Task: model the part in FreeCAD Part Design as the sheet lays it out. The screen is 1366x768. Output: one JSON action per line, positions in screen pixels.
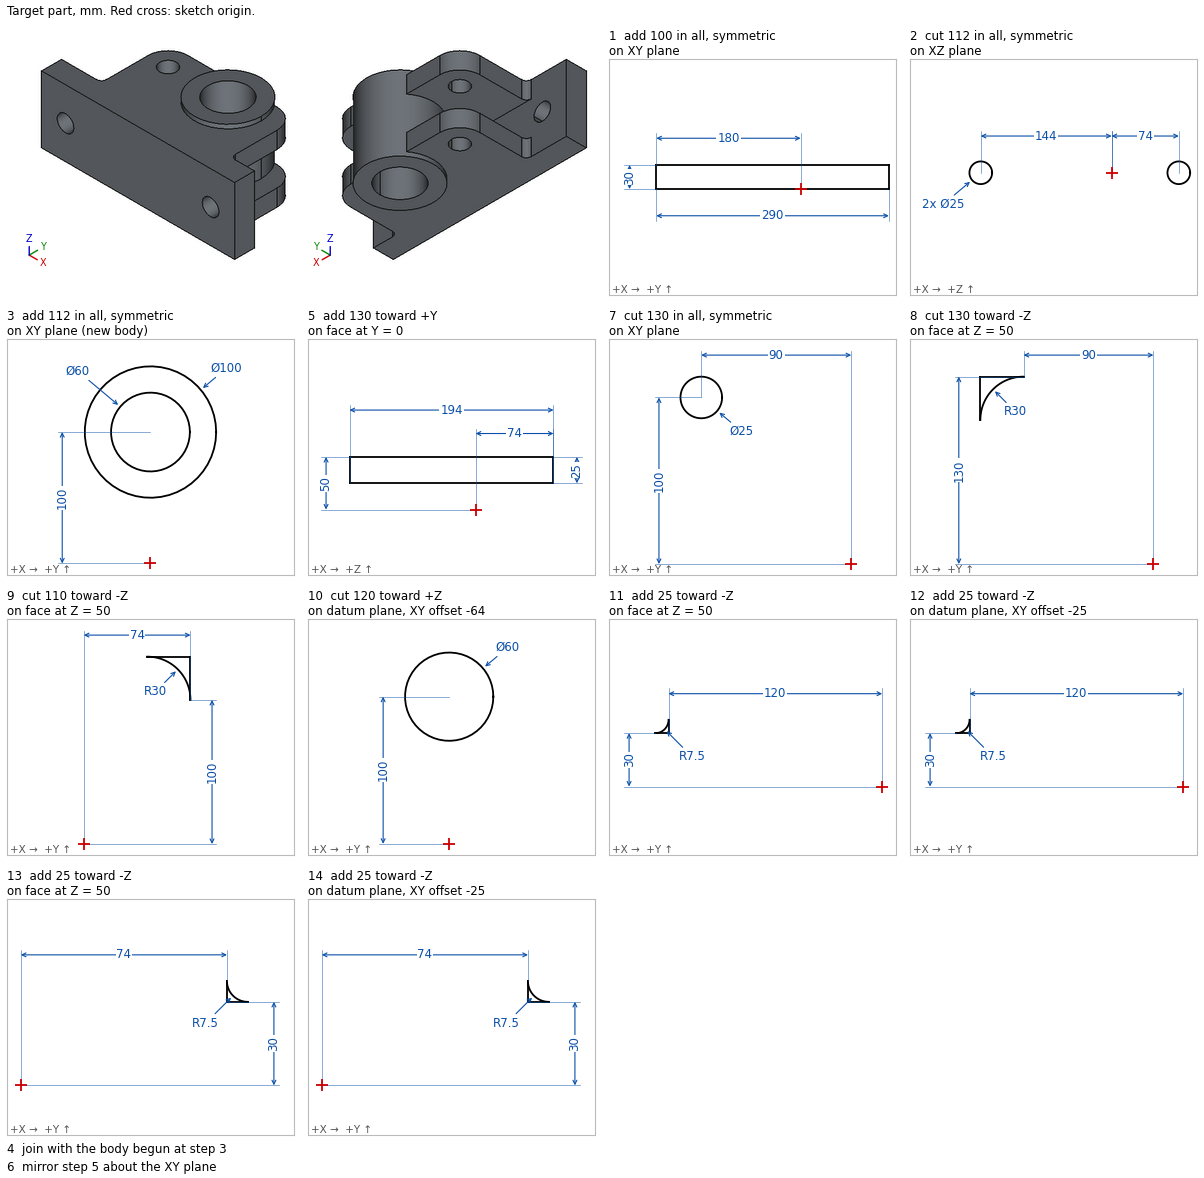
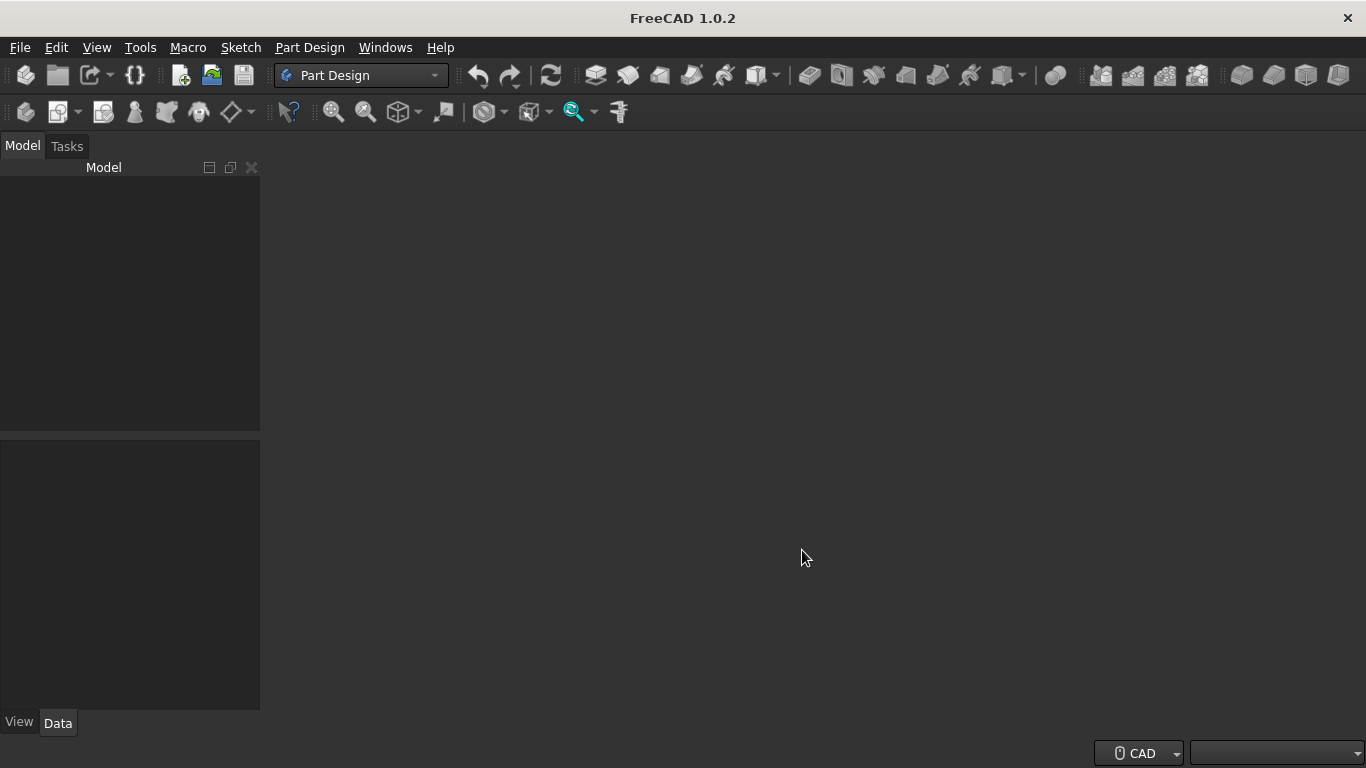
{"action": "left_click", "coordinate": [180, 76]}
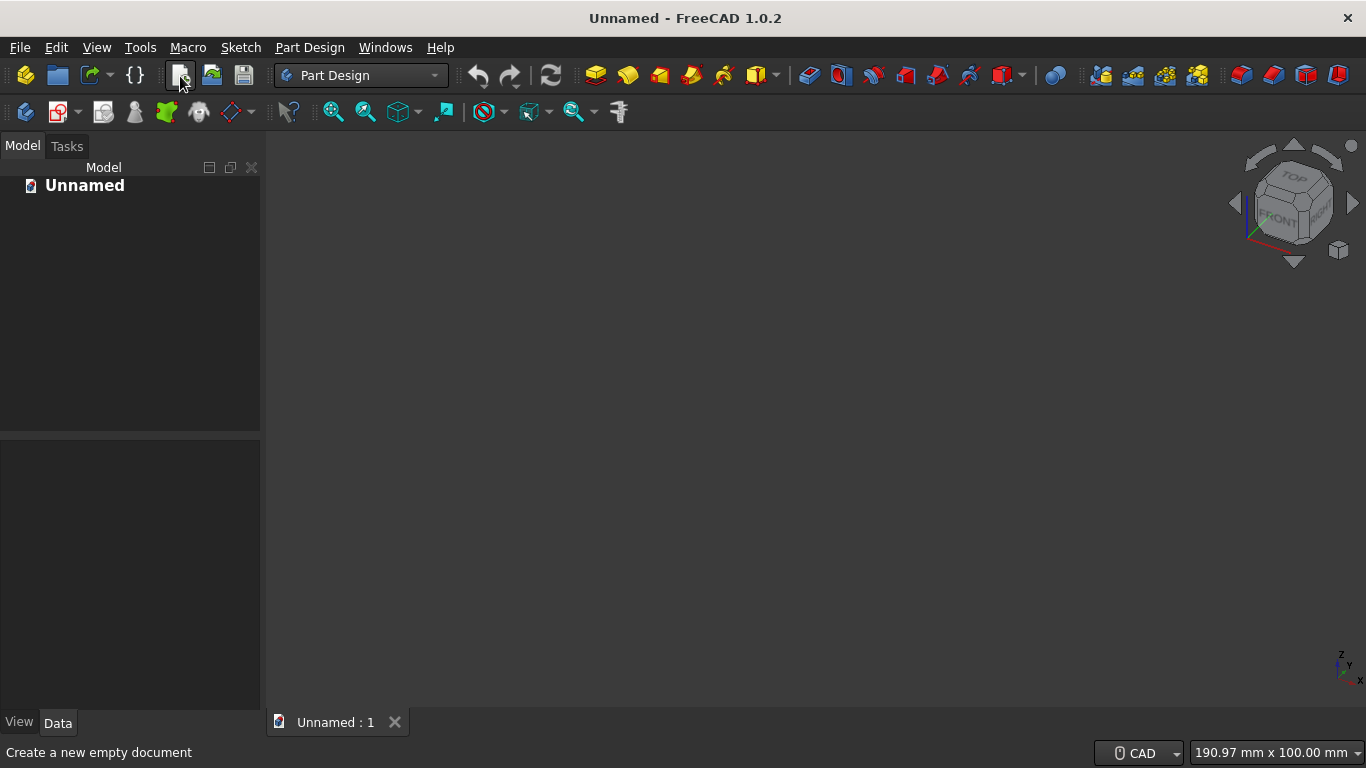
{"action": "left_click", "coordinate": [58, 112]}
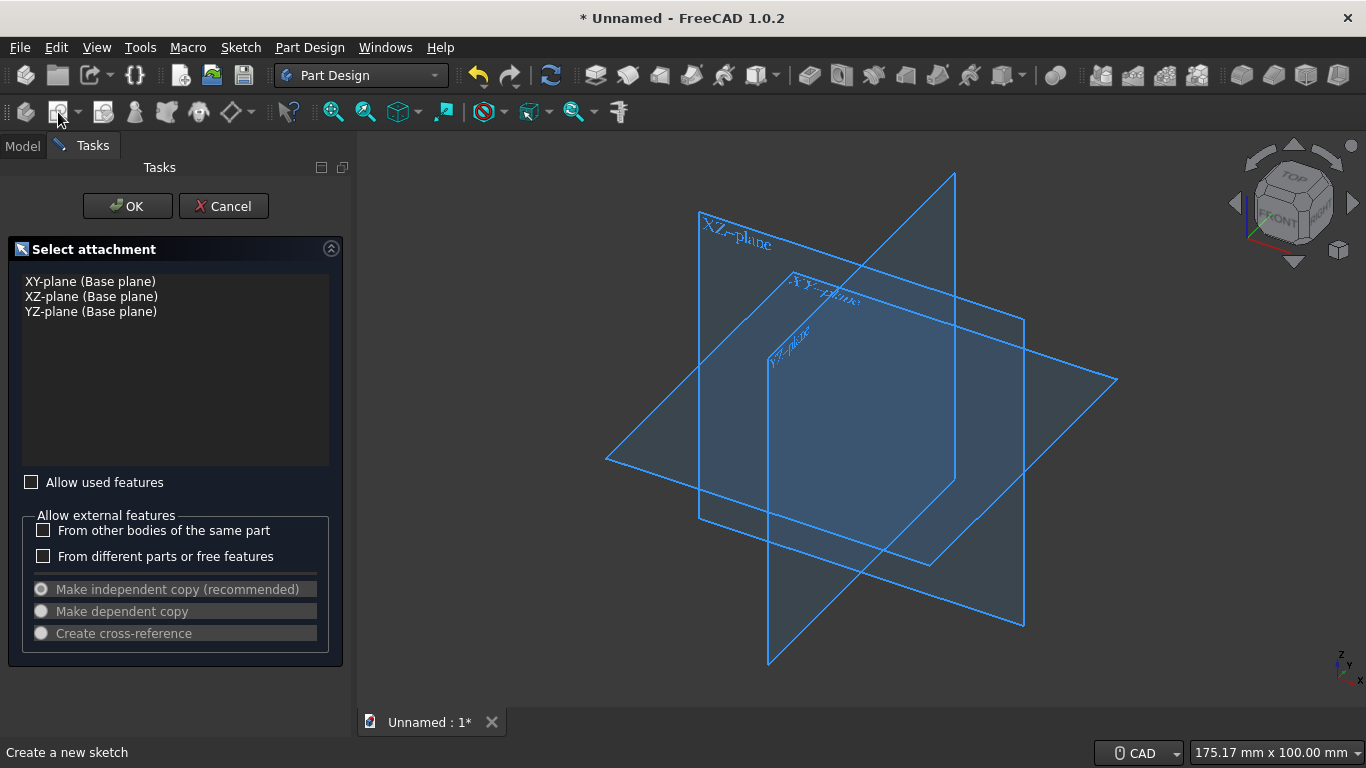
{"action": "left_click", "coordinate": [82, 282]}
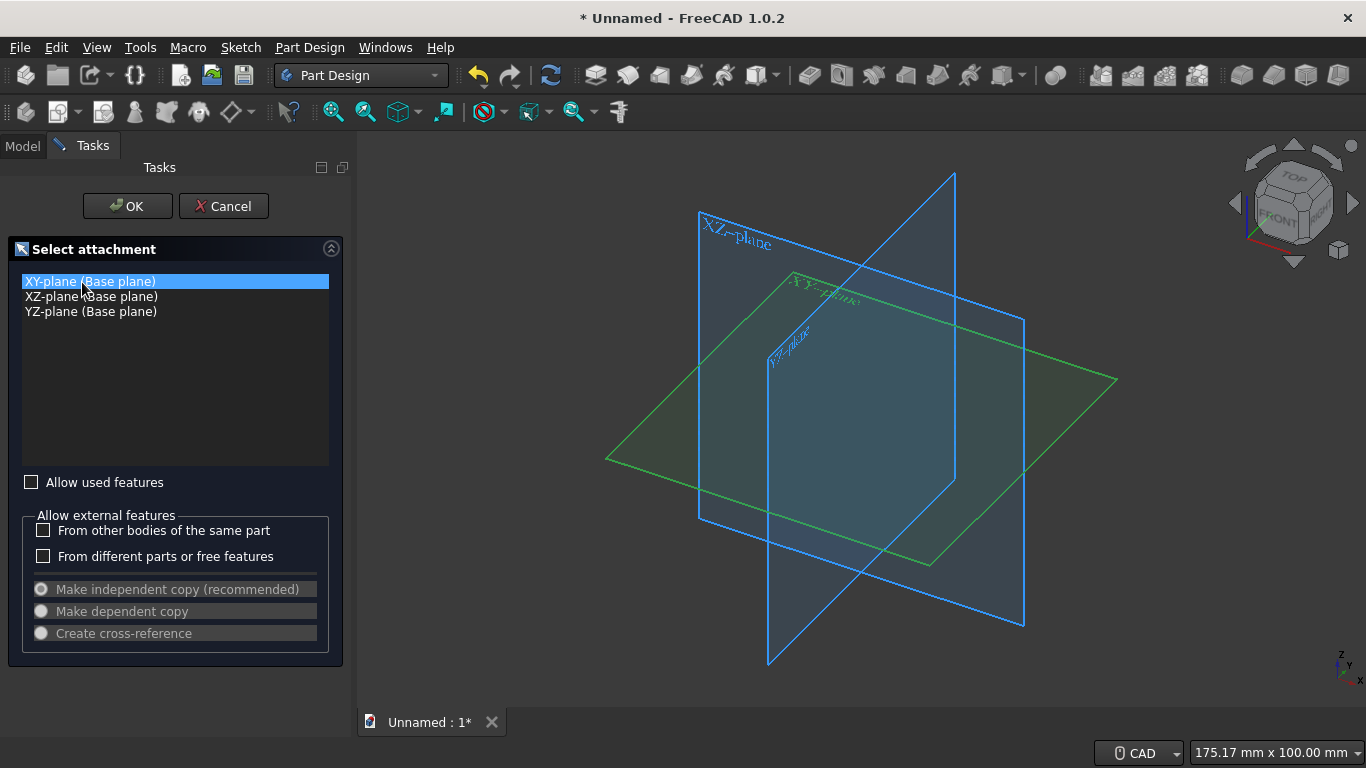
{"action": "left_click", "coordinate": [128, 206]}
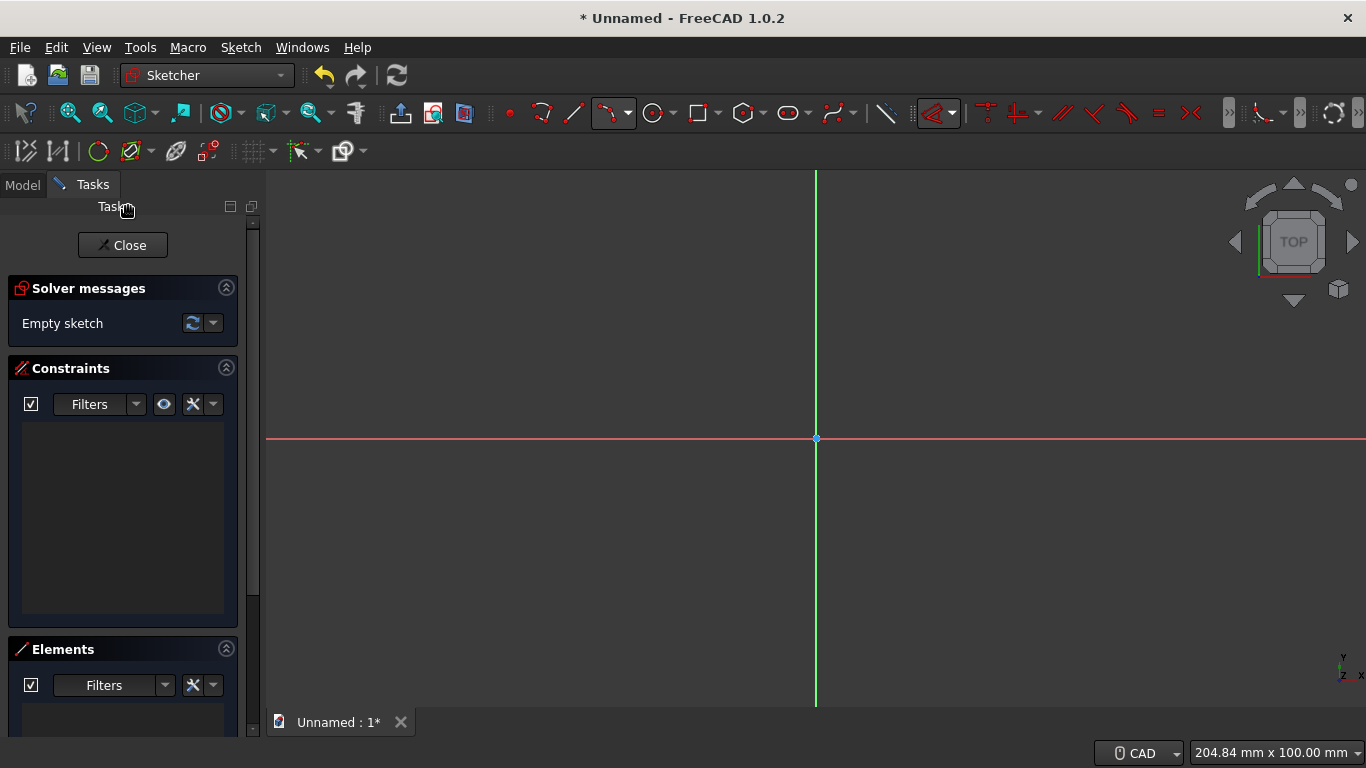
{"action": "scroll", "coordinate": [845, 504], "scroll_direction": "down", "scroll_amount": 4}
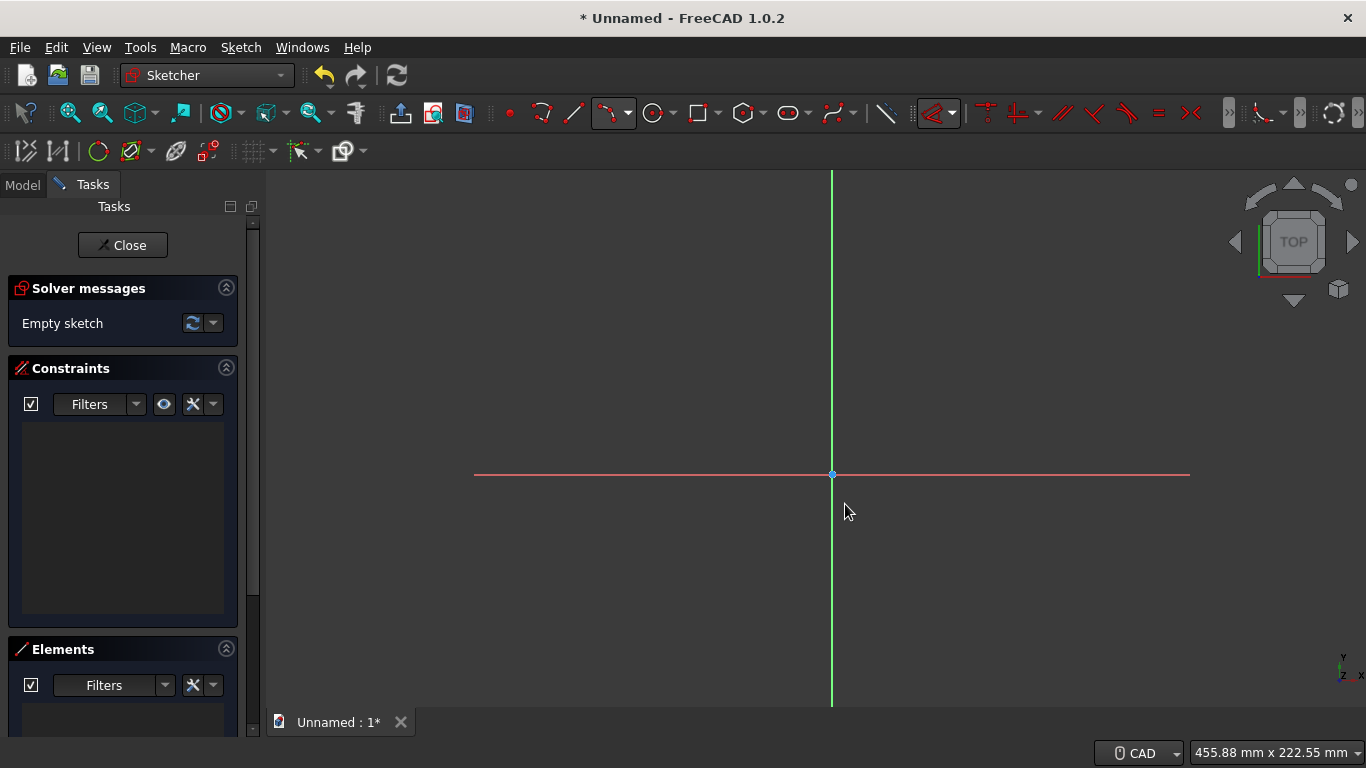
{"action": "left_click", "coordinate": [698, 114]}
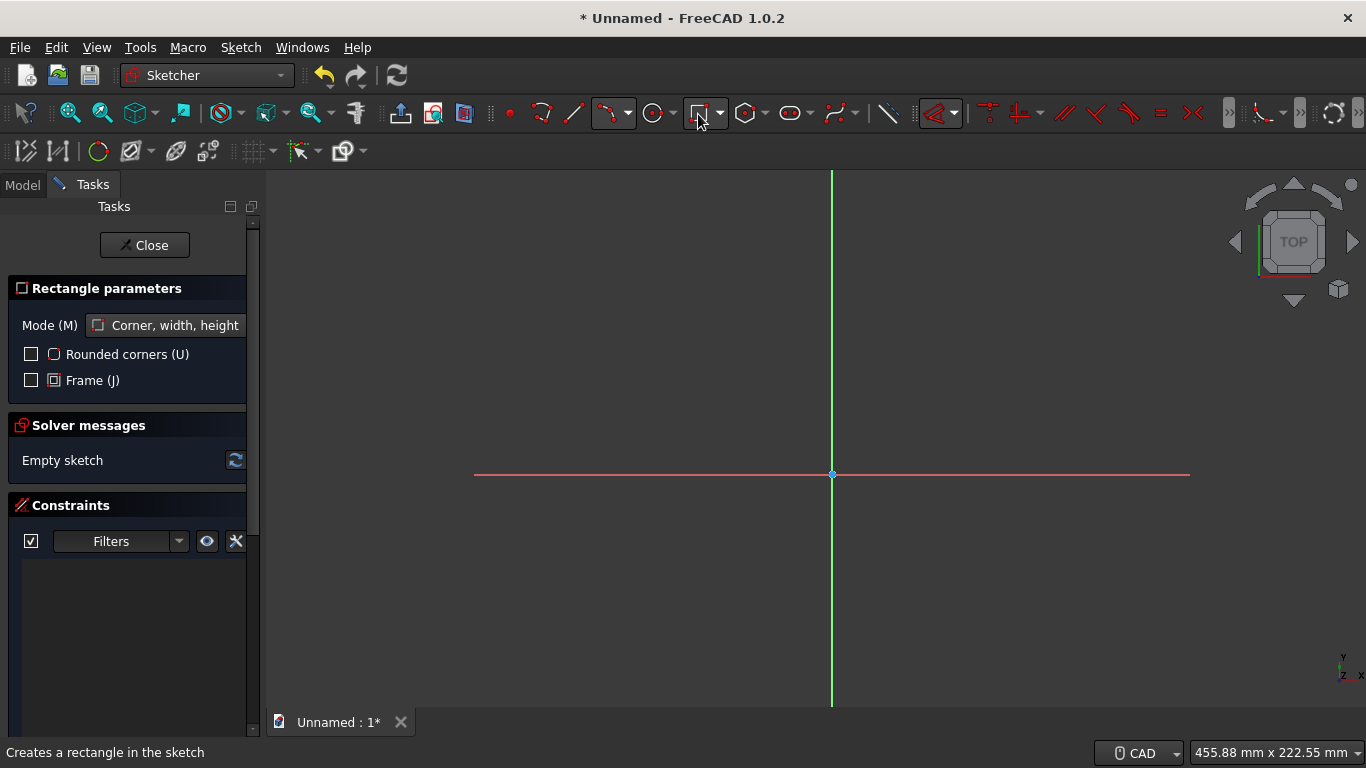
{"action": "left_click", "coordinate": [398, 403]}
{"action": "left_click", "coordinate": [1098, 475]}
{"action": "key", "text": "Escape"}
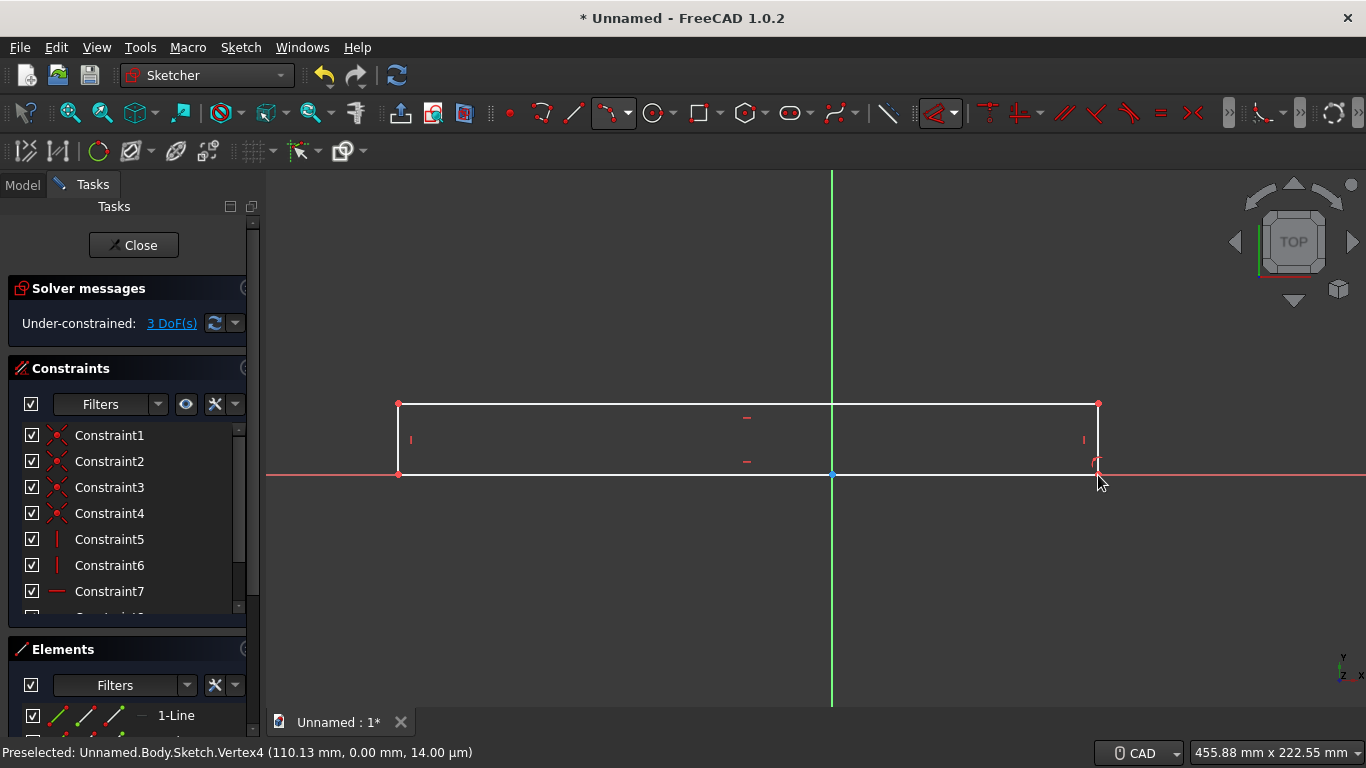
{"action": "left_click", "coordinate": [934, 114]}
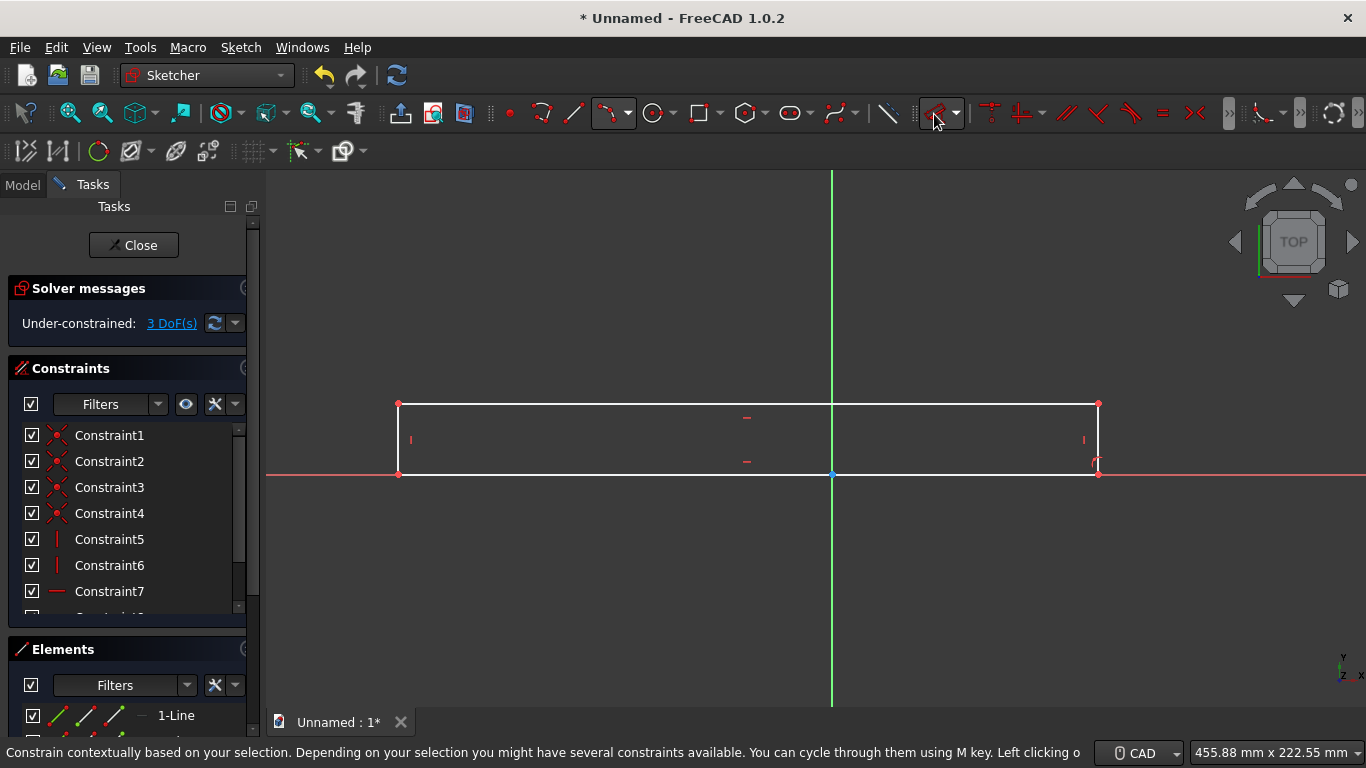
{"action": "left_click", "coordinate": [398, 425]}
{"action": "left_click", "coordinate": [364, 439]}